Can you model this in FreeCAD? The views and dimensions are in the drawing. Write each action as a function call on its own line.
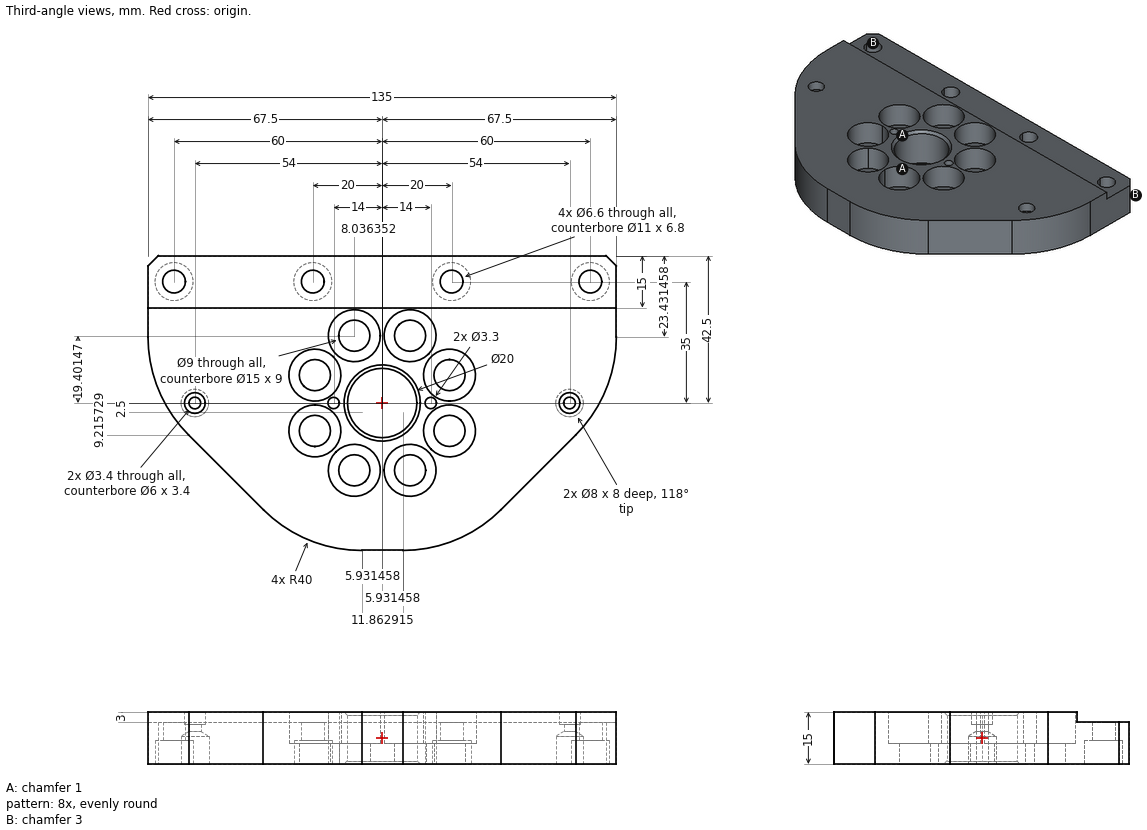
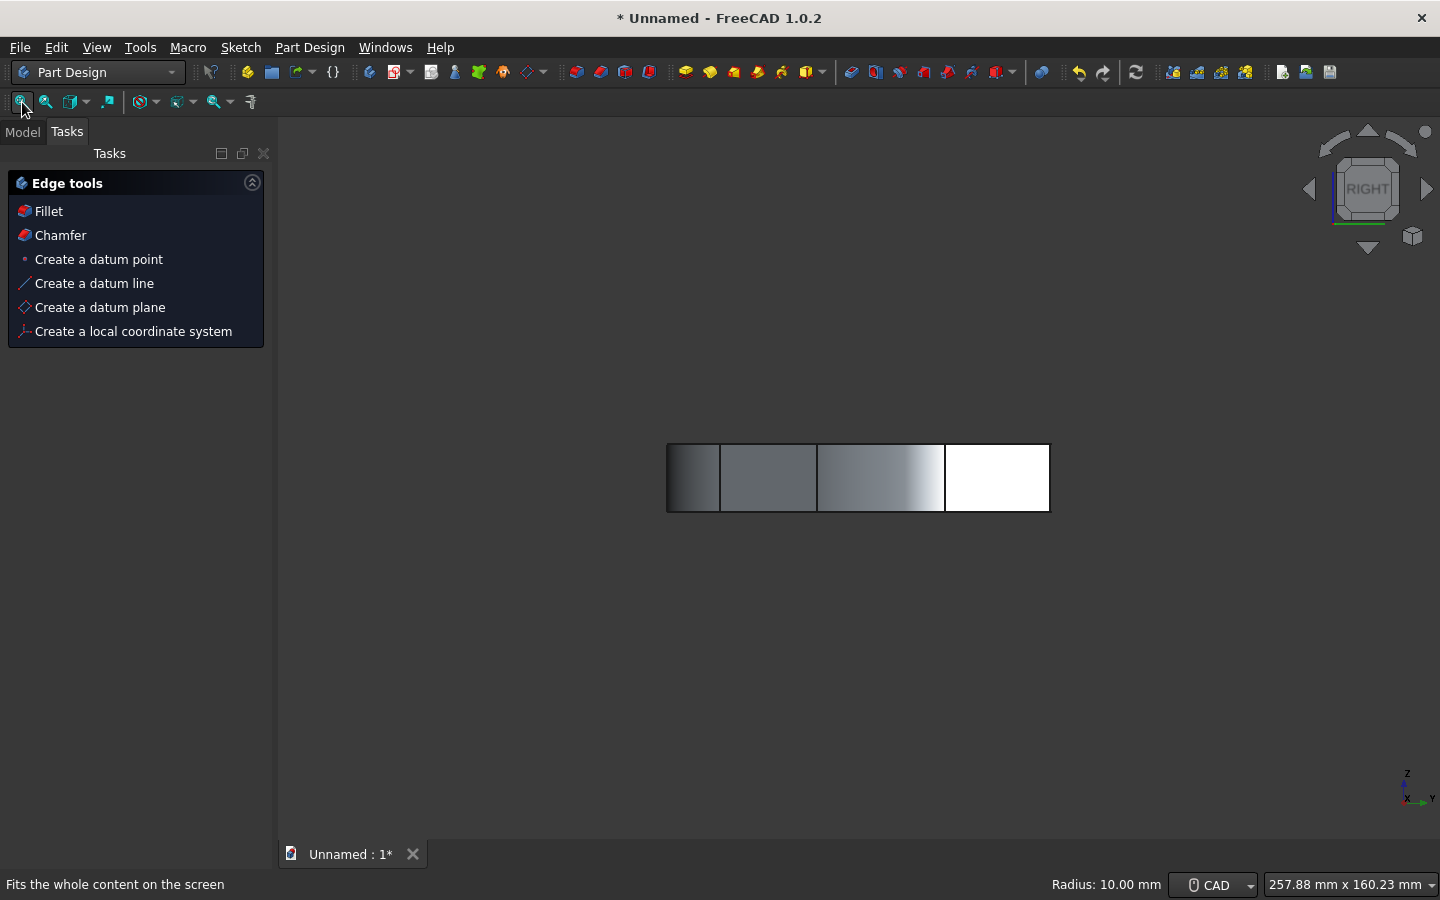
key(5)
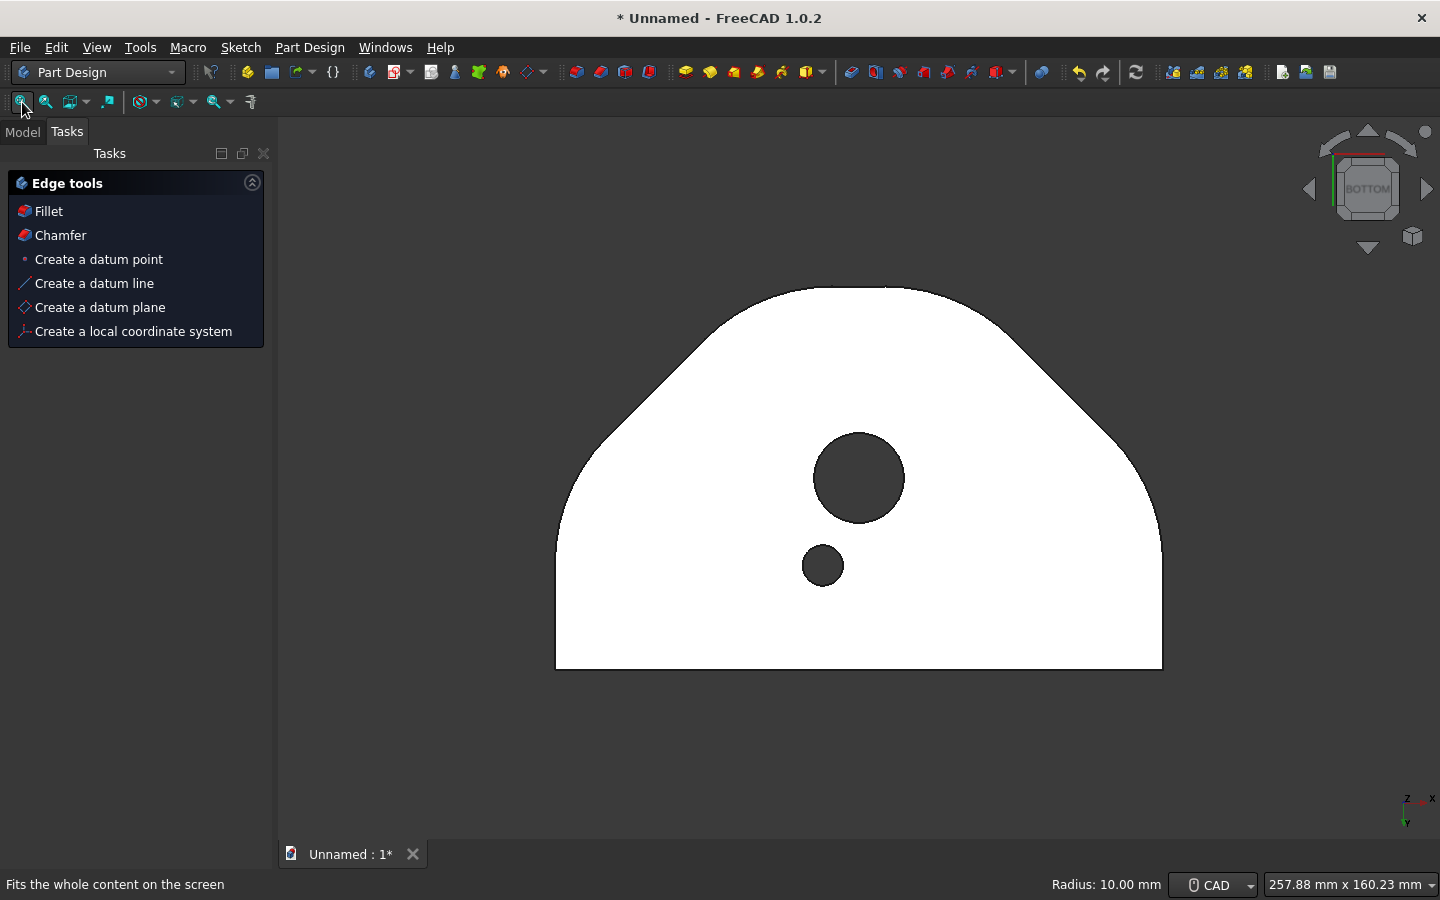
click(814, 477, ctrl)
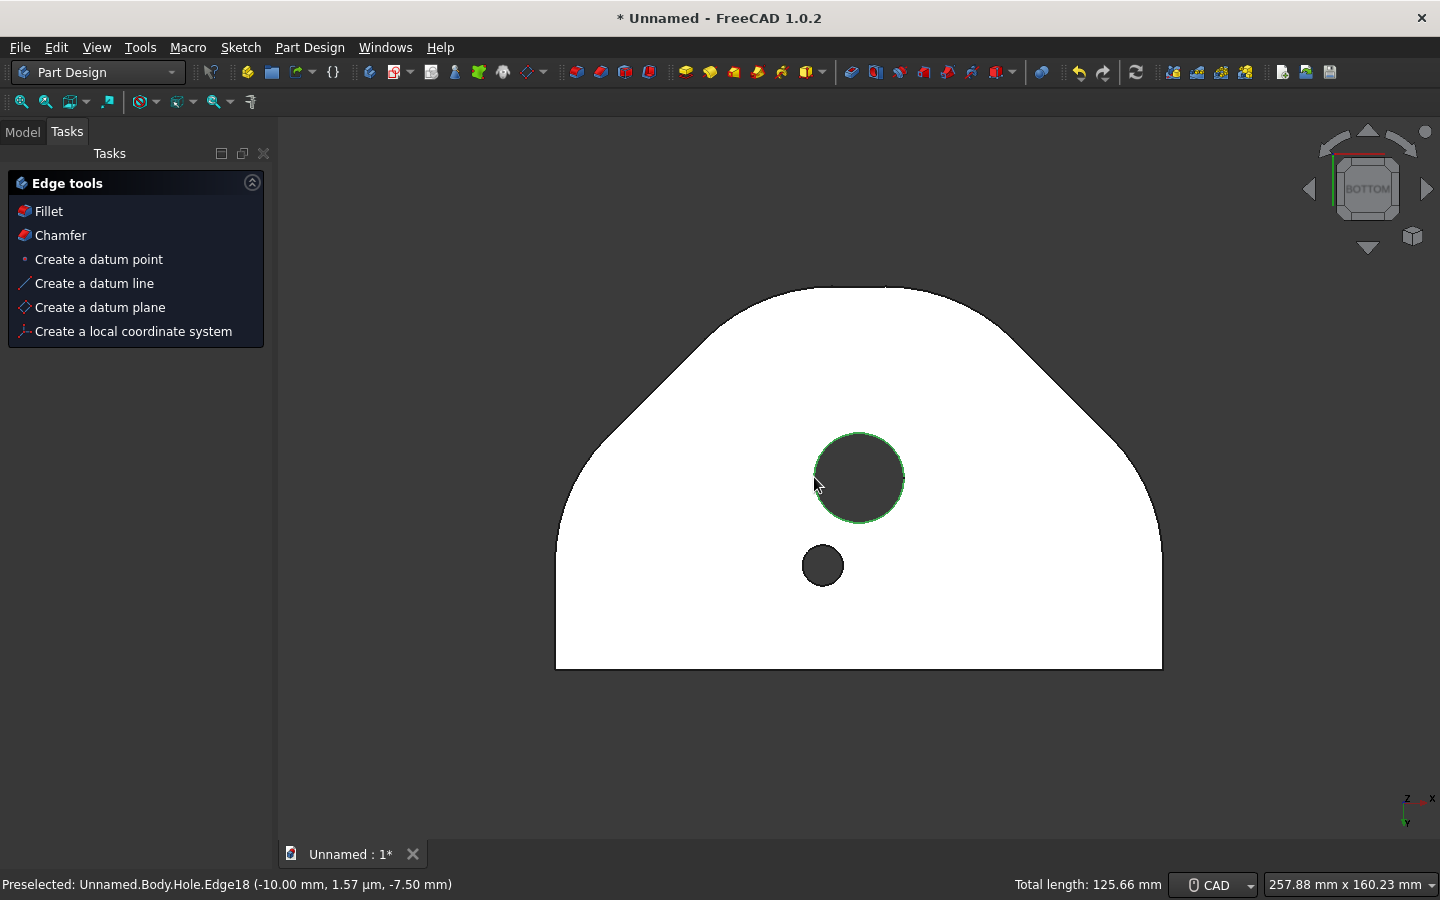
click(602, 72)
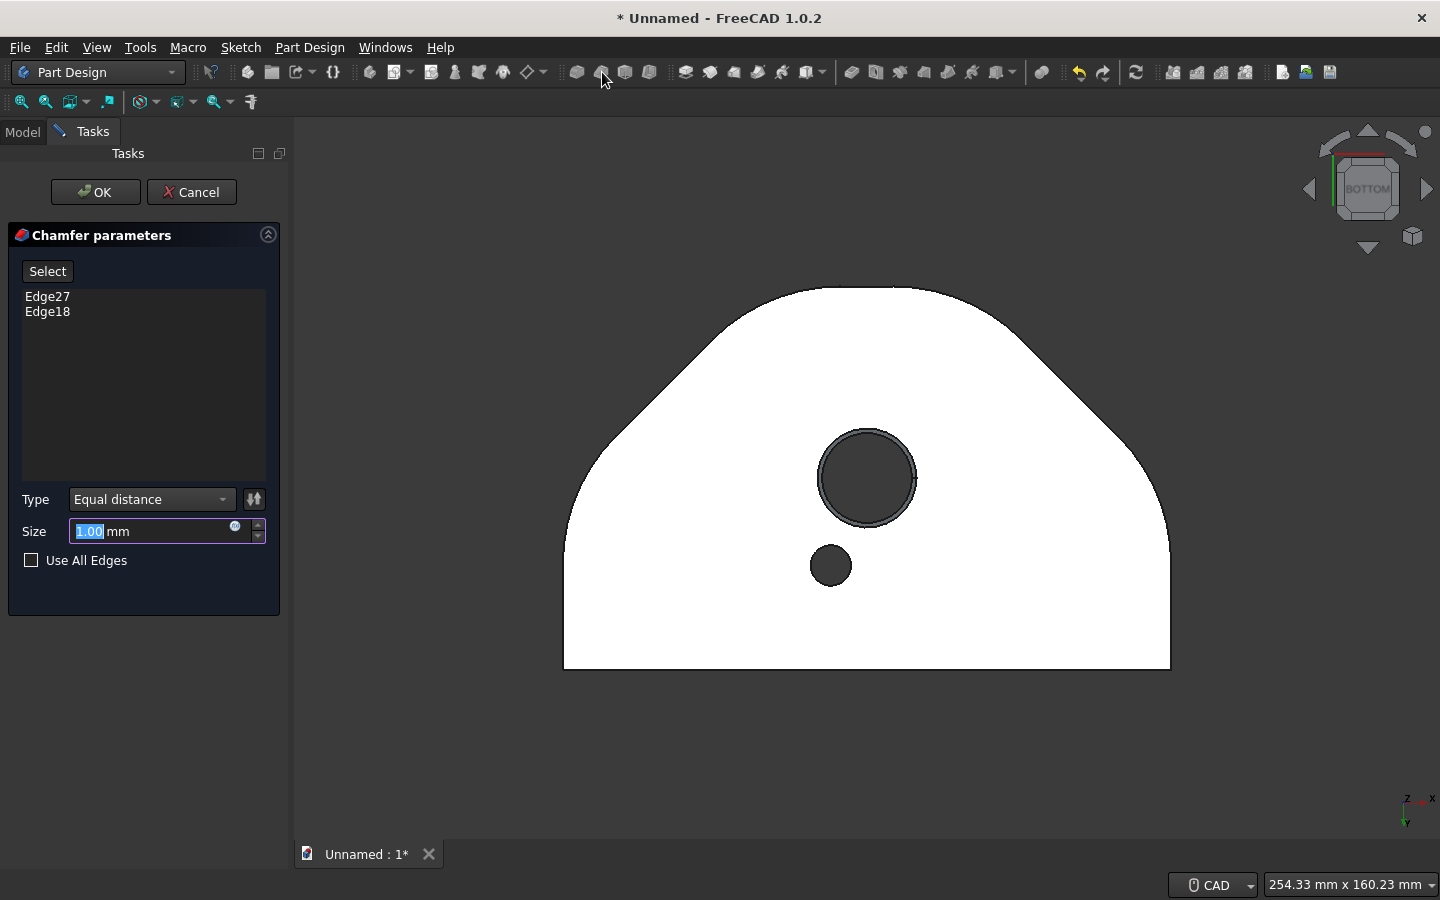
text(1)
key(Tab)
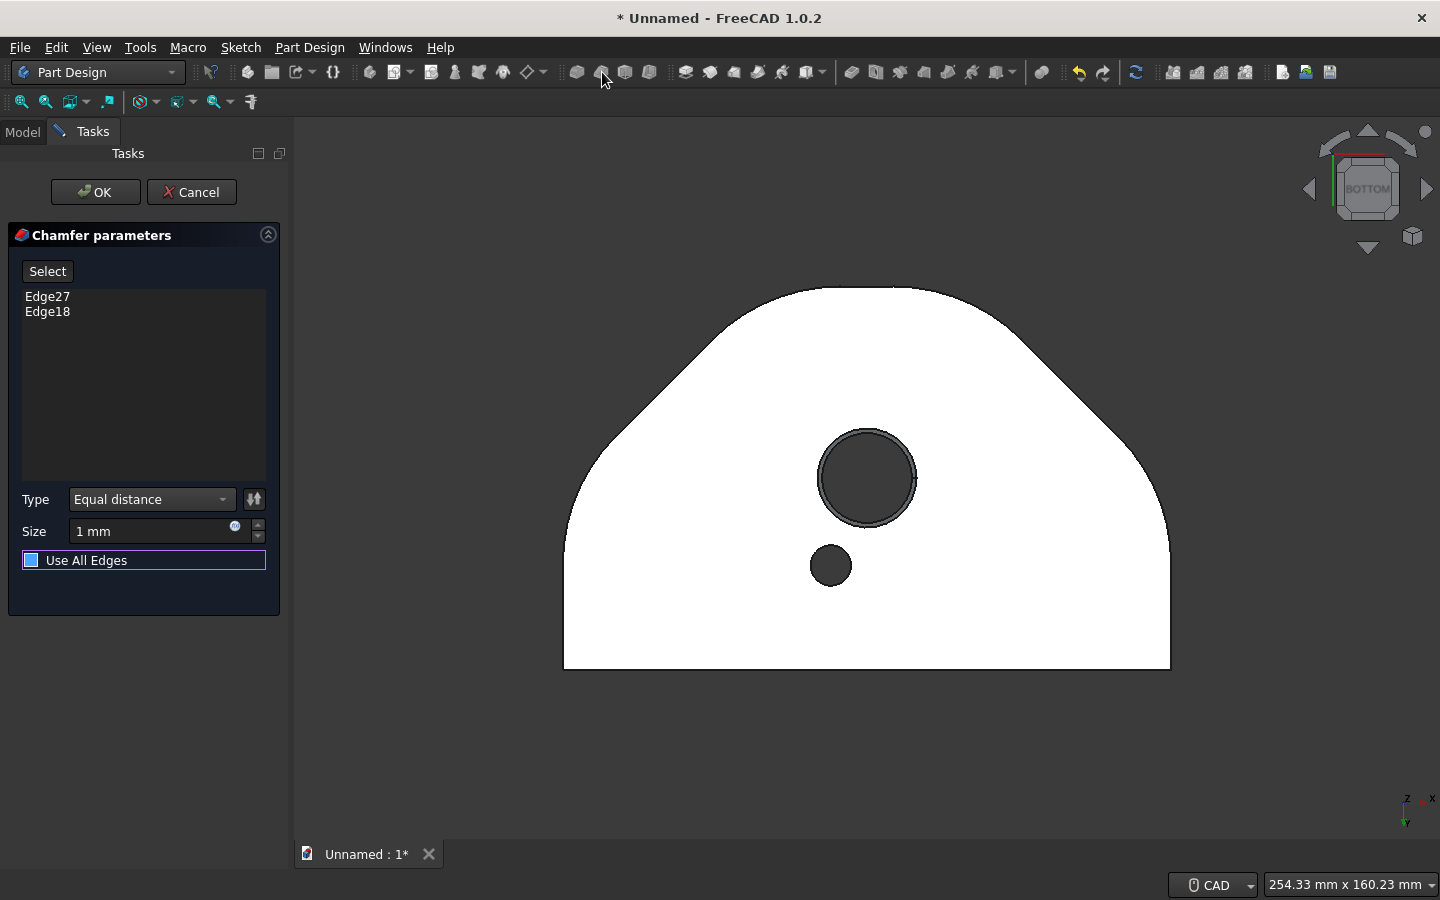
click(96, 192)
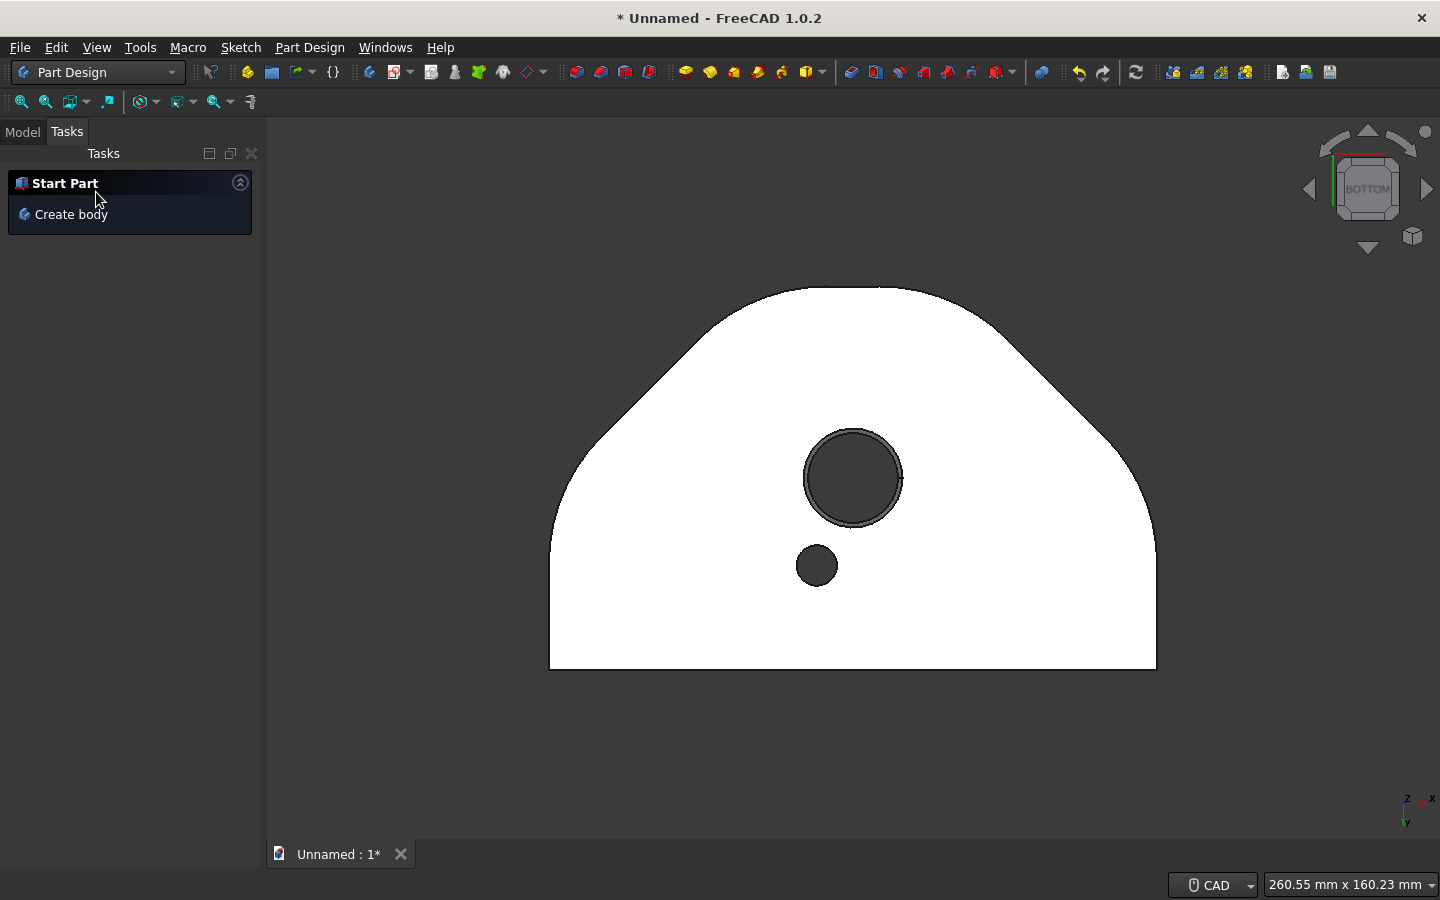
click(23, 131)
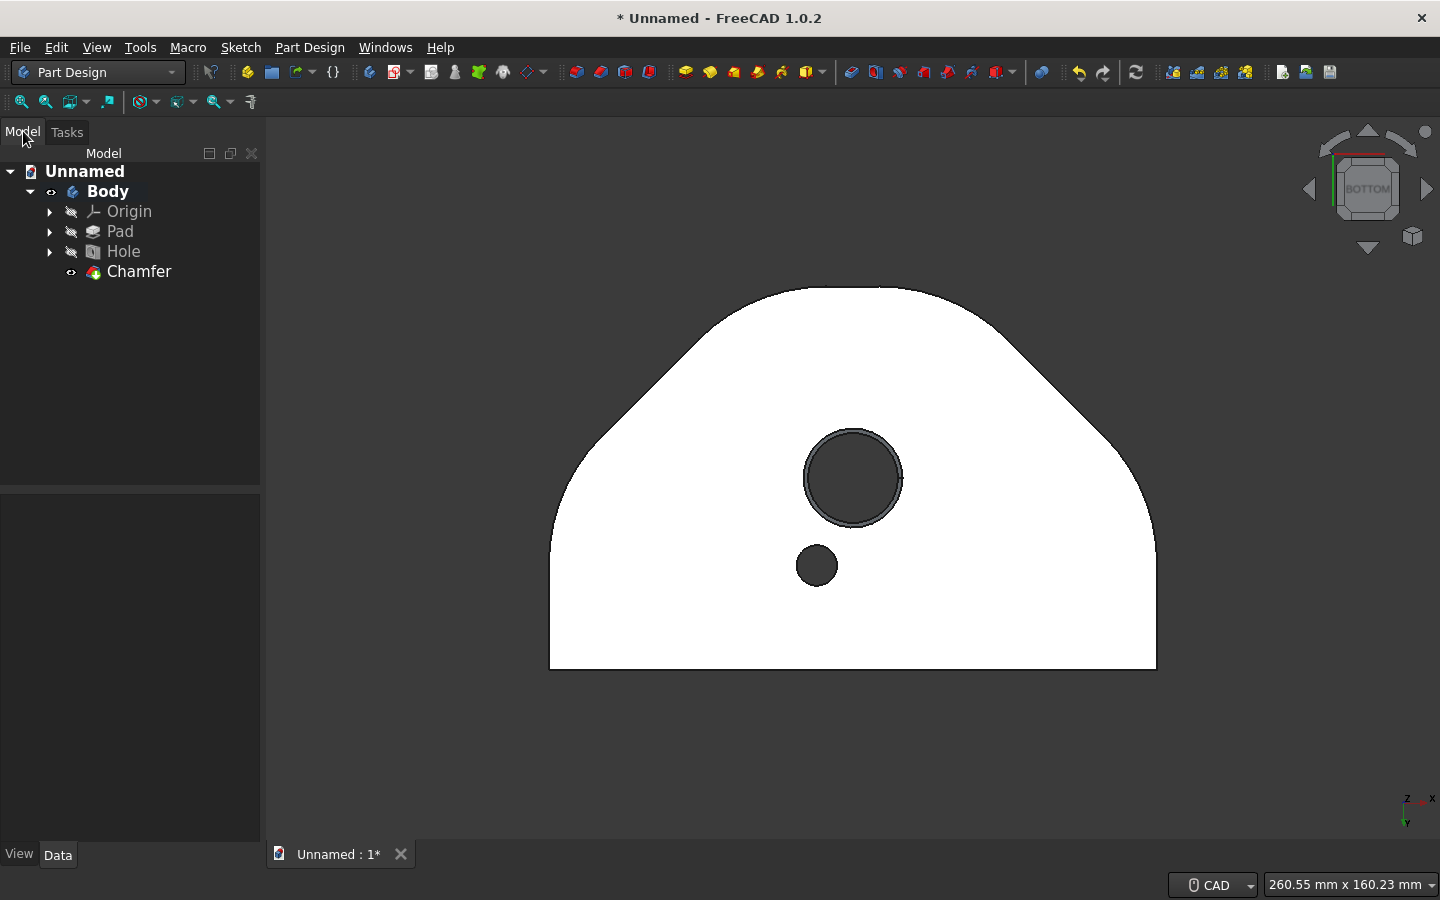
click(116, 252)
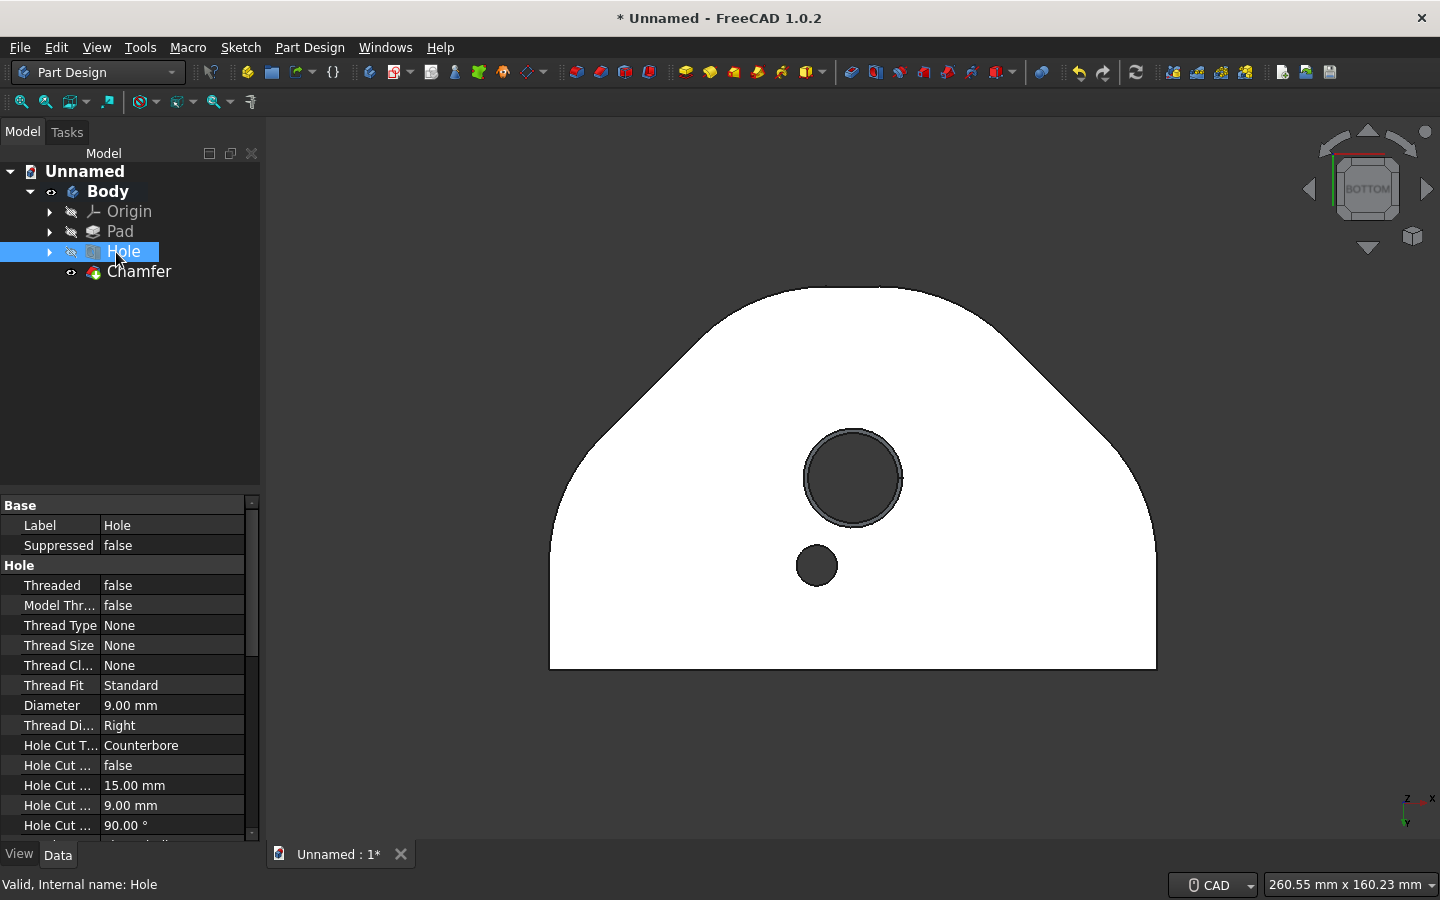
click(1222, 72)